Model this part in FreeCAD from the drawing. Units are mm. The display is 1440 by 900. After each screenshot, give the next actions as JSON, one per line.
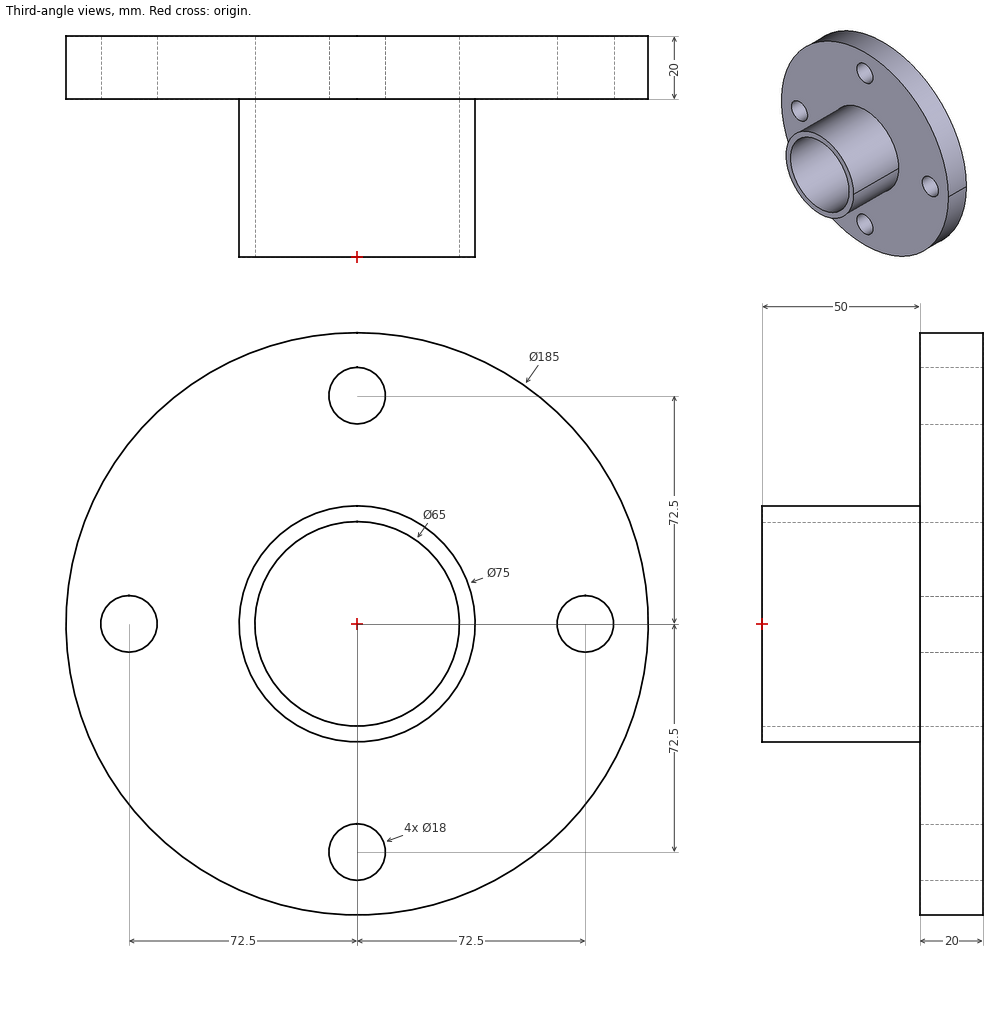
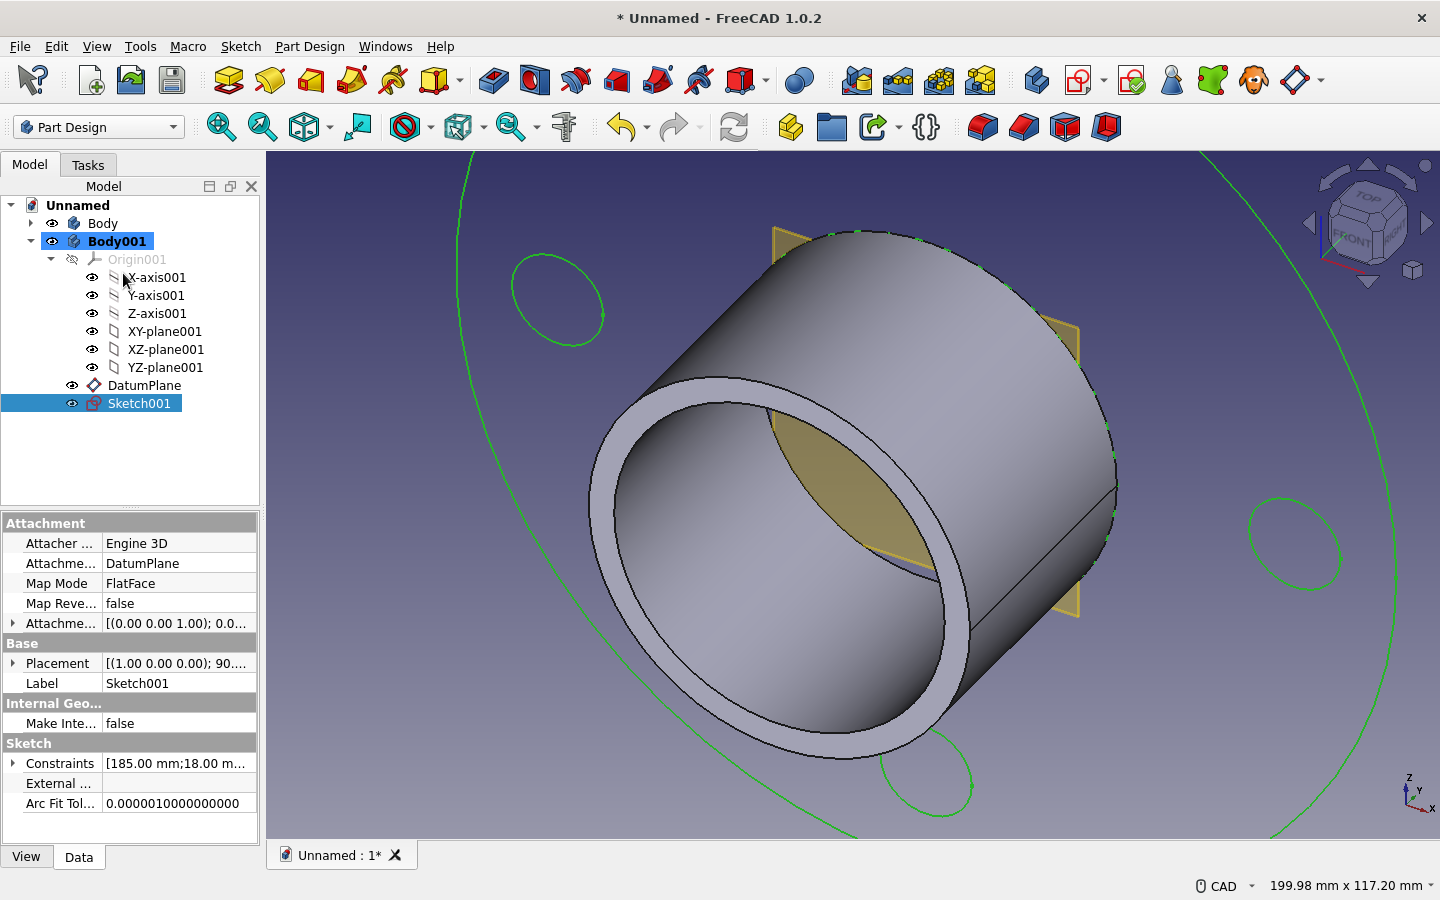
{"action": "left_click", "coordinate": [229, 80]}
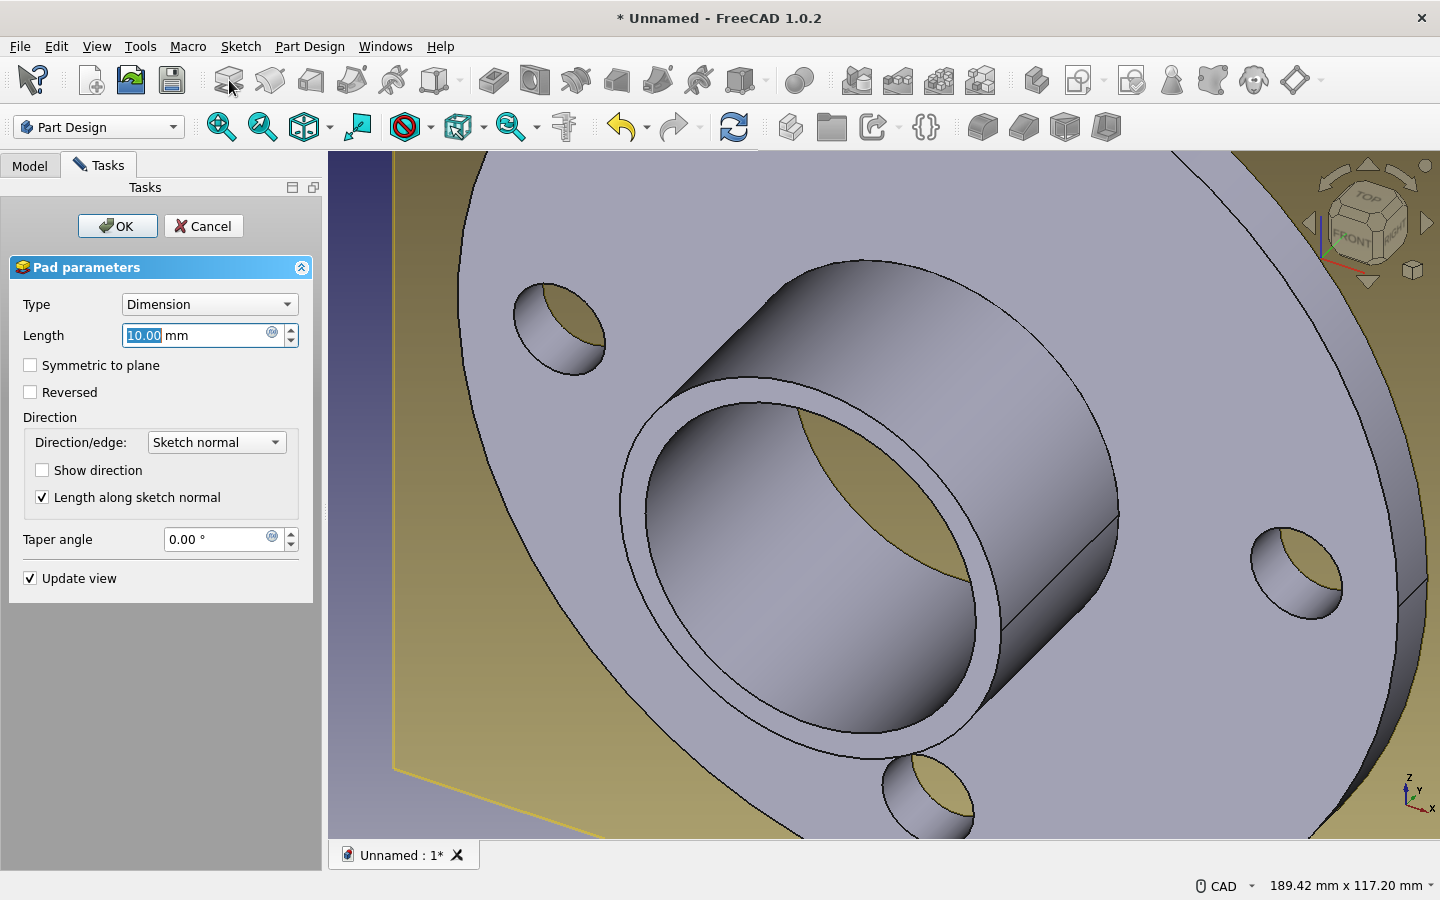
{"action": "type", "text": "20"}
{"action": "key", "text": "Tab"}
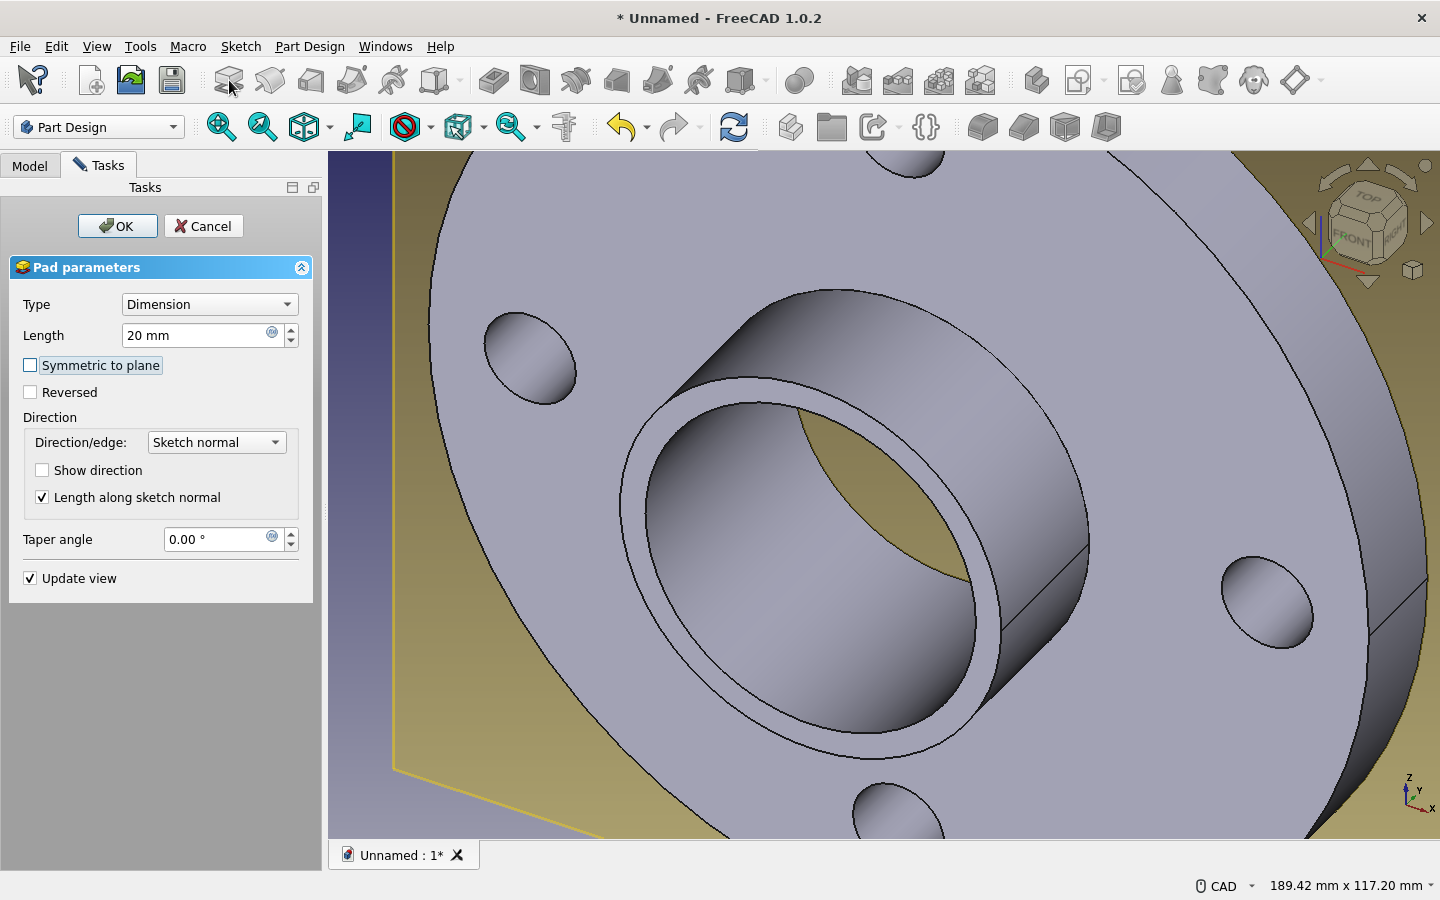
{"action": "left_click", "coordinate": [31, 392]}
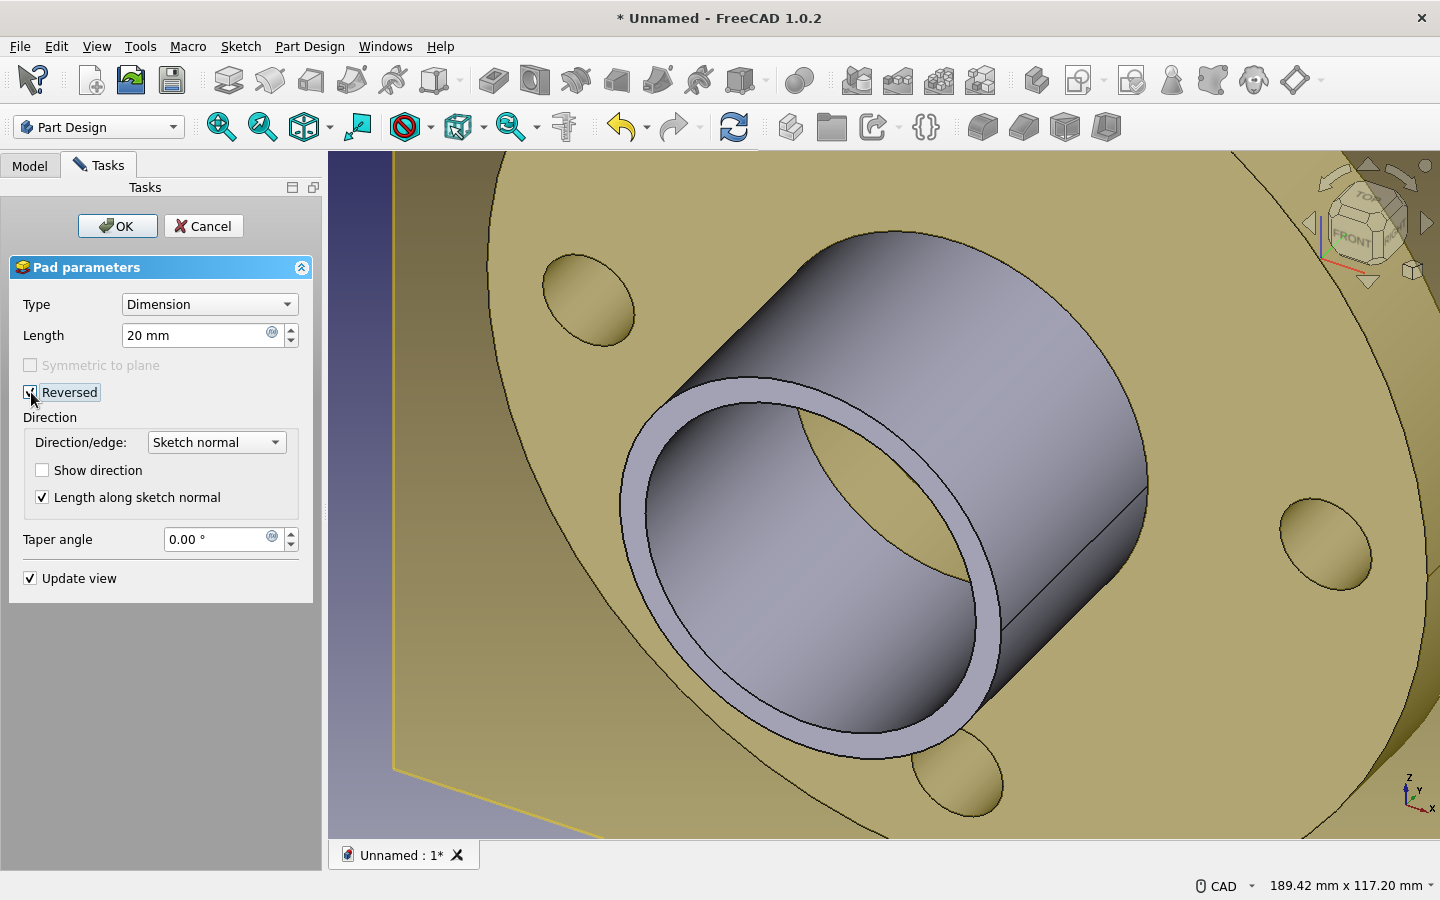
{"action": "left_click", "coordinate": [118, 226]}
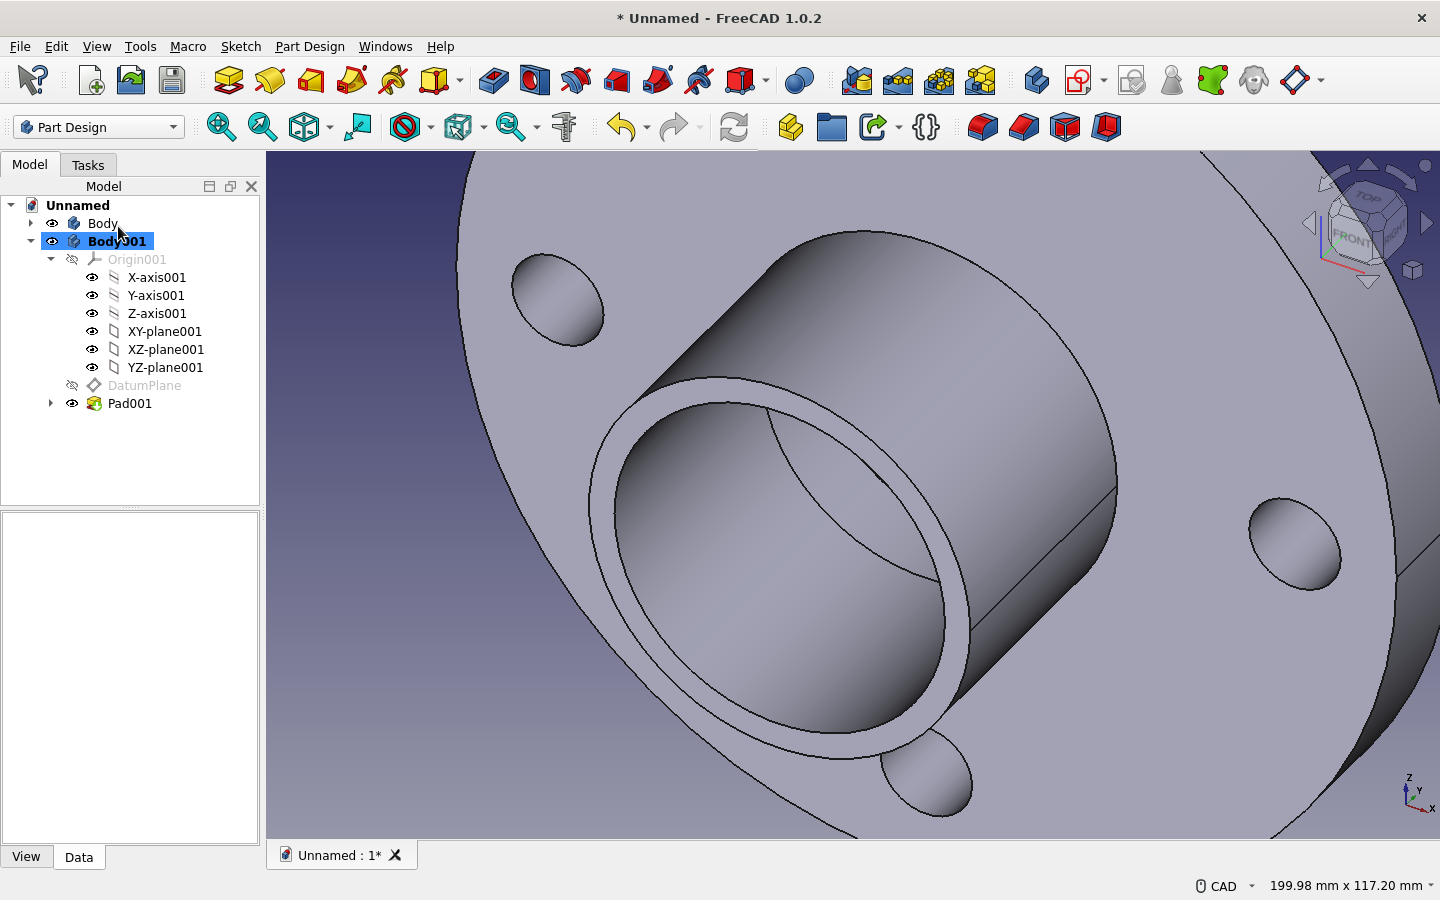
{"action": "left_click", "coordinate": [222, 128]}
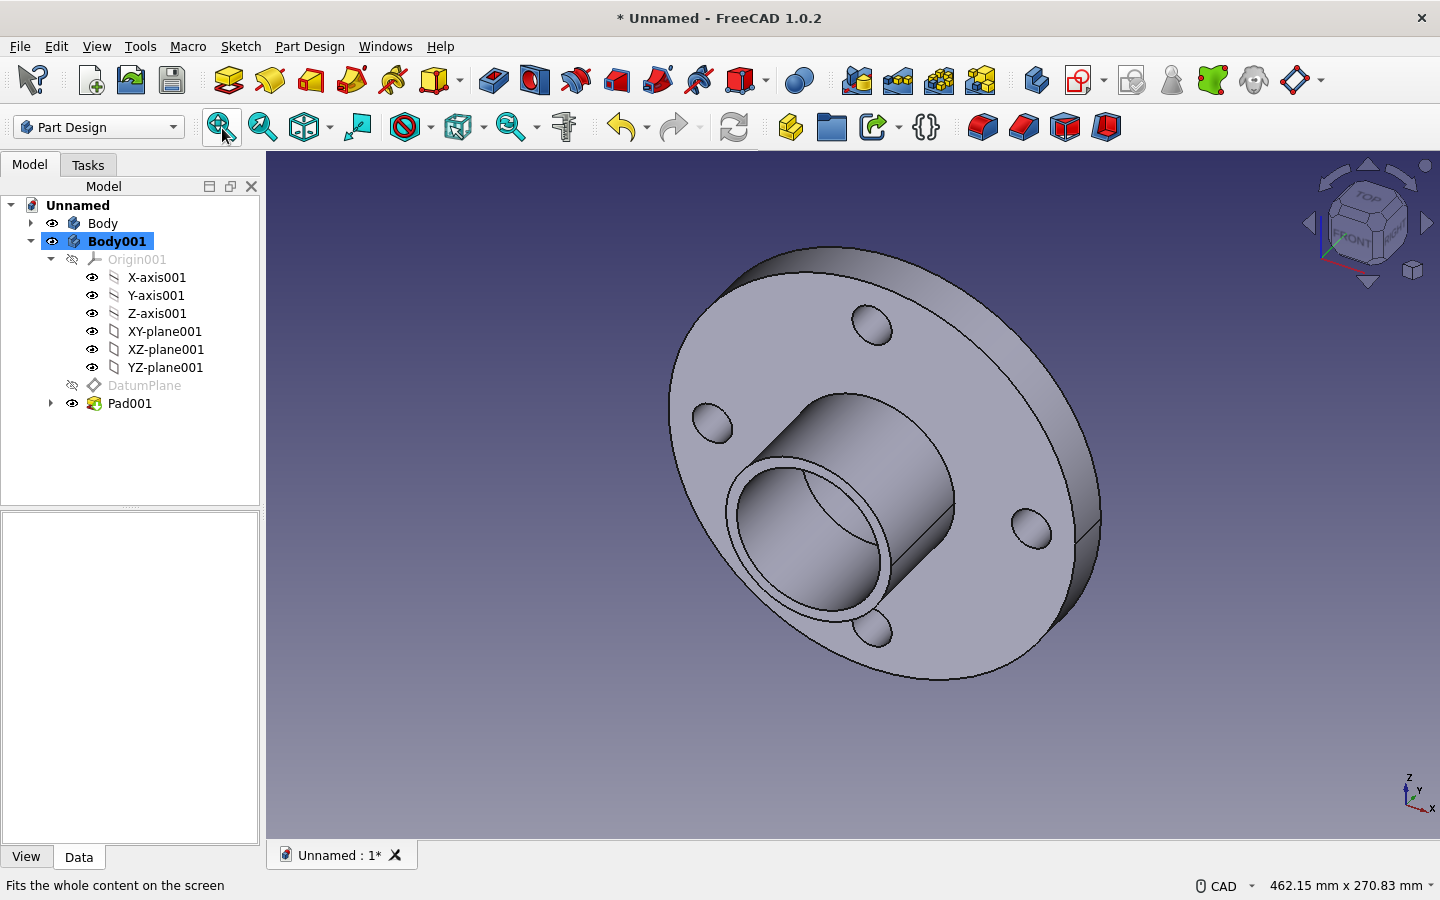
{"action": "double_click", "coordinate": [97, 223]}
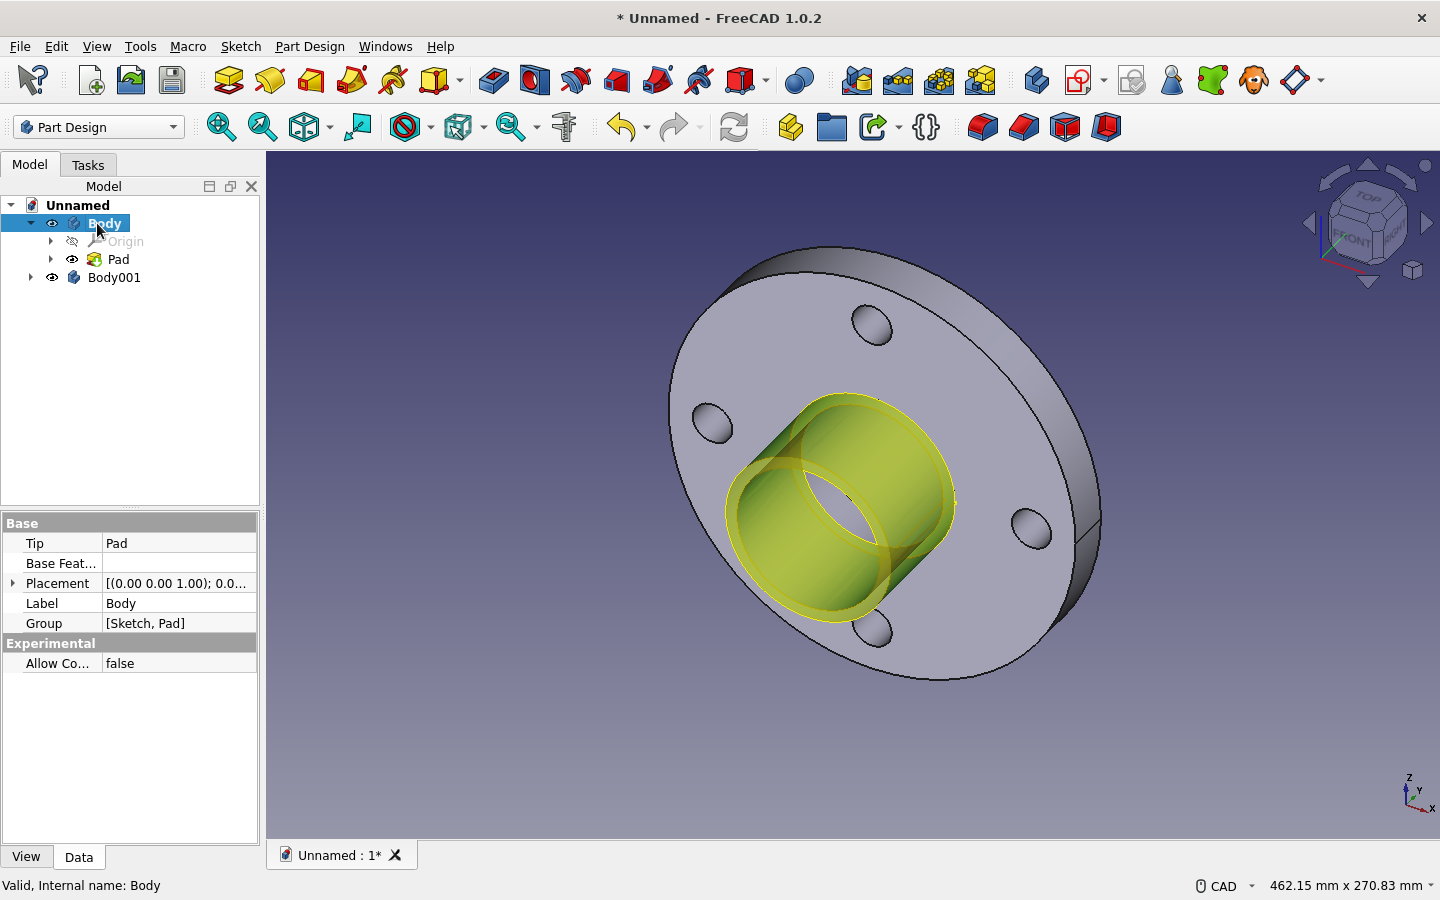
{"action": "left_click", "coordinate": [97, 223]}